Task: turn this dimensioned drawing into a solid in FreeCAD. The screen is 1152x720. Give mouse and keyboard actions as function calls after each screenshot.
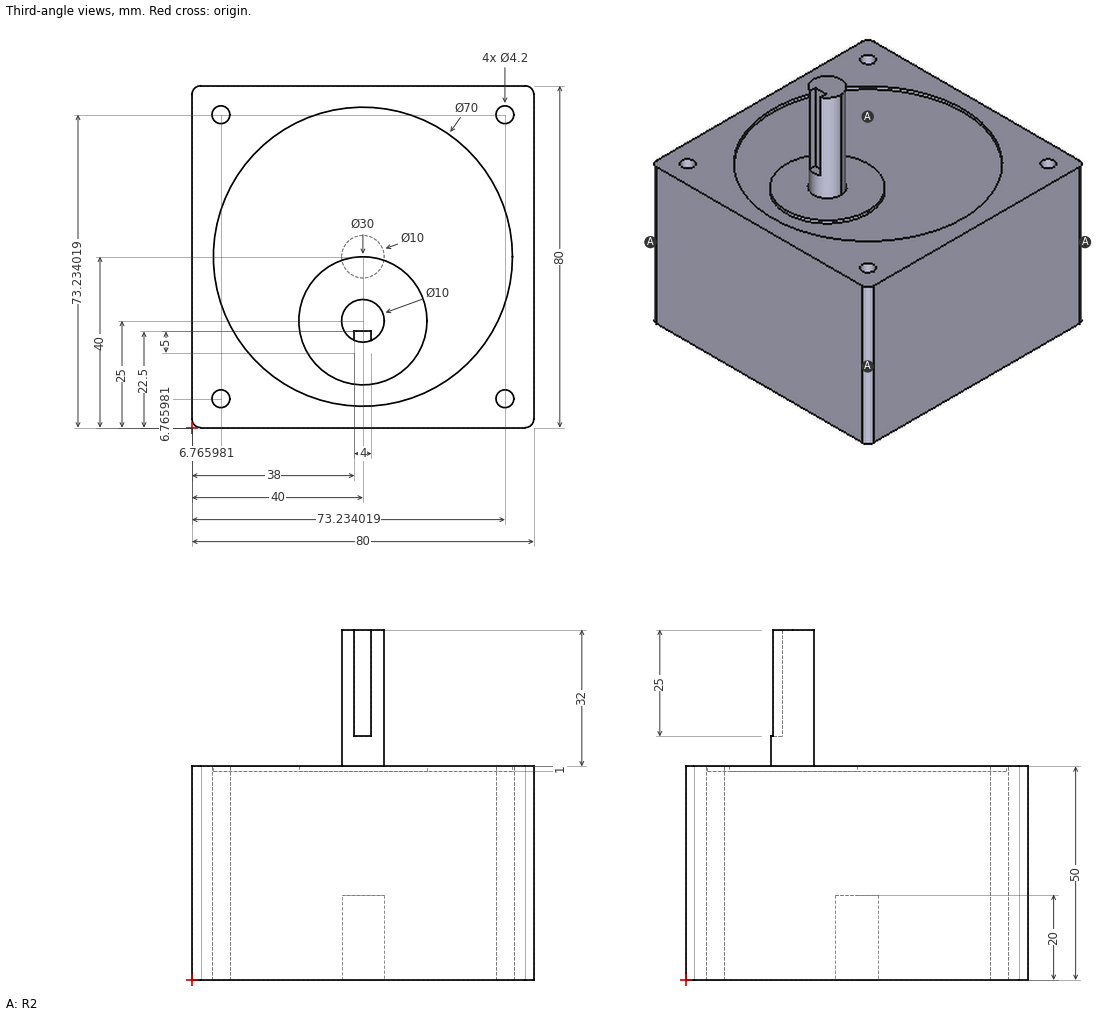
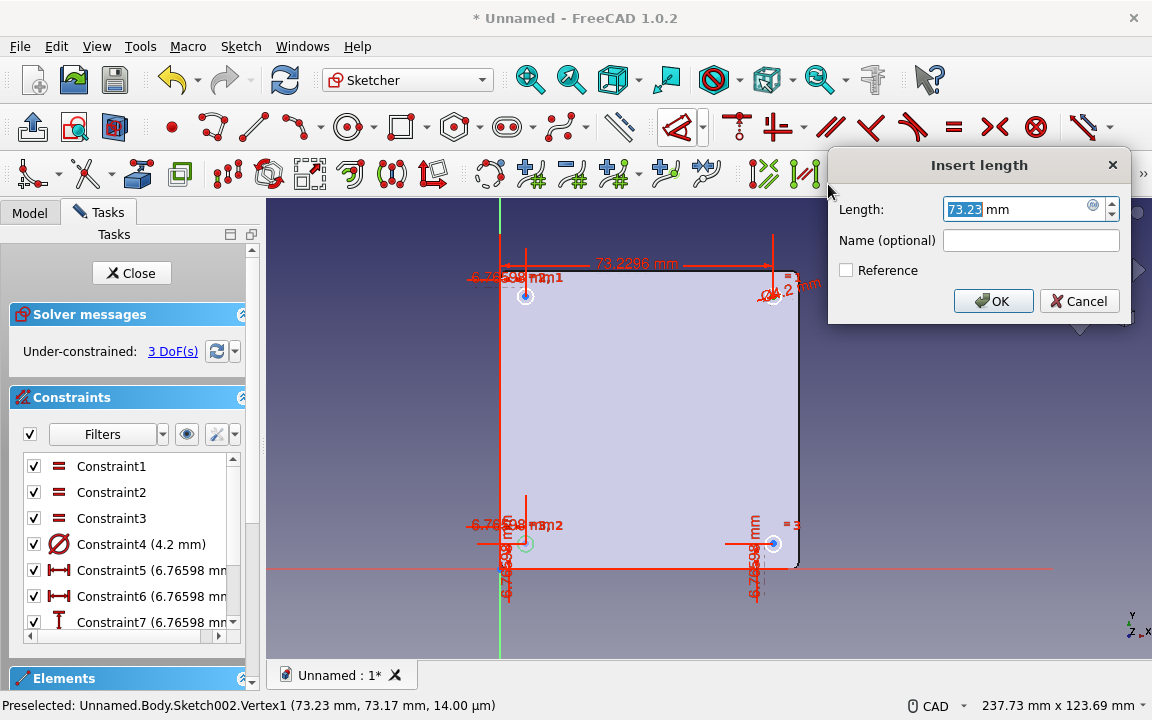
text(73.234019)
key(Return)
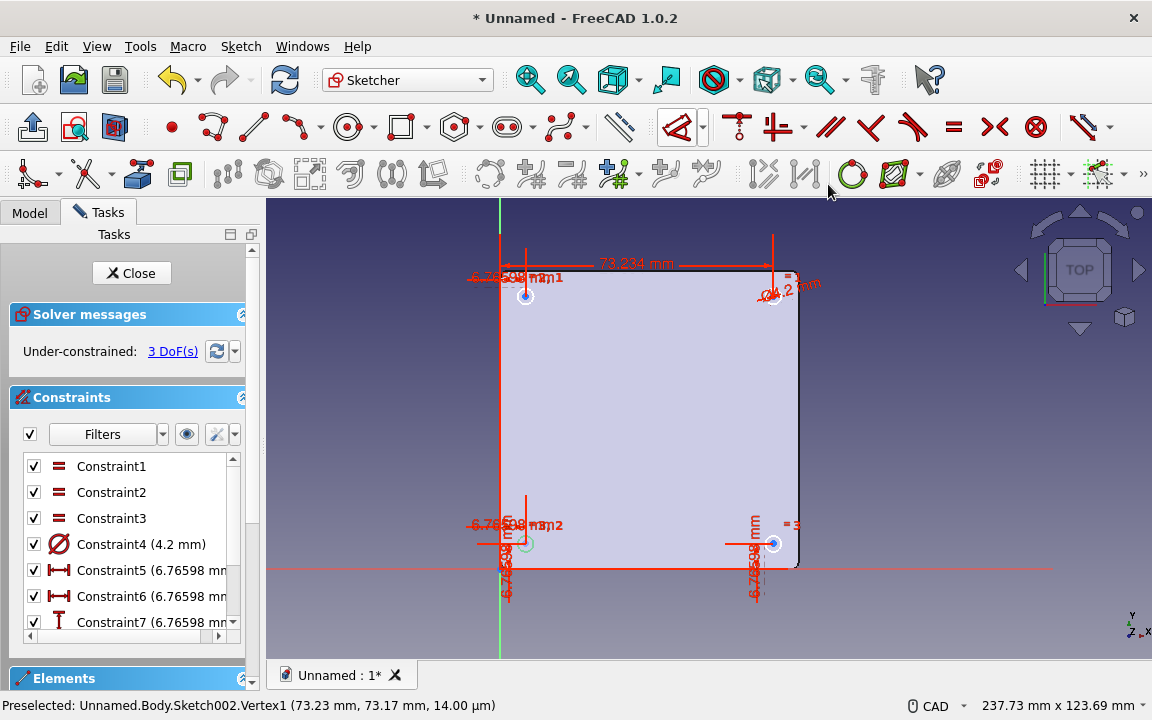
click(773, 296)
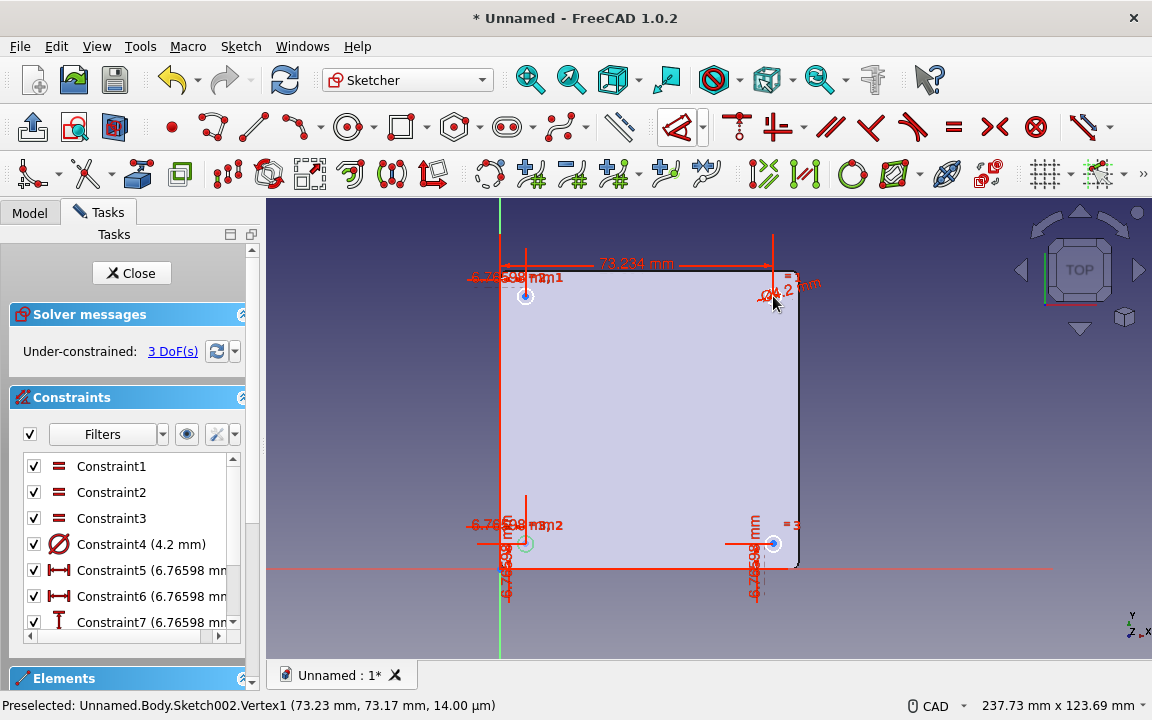
click(702, 128)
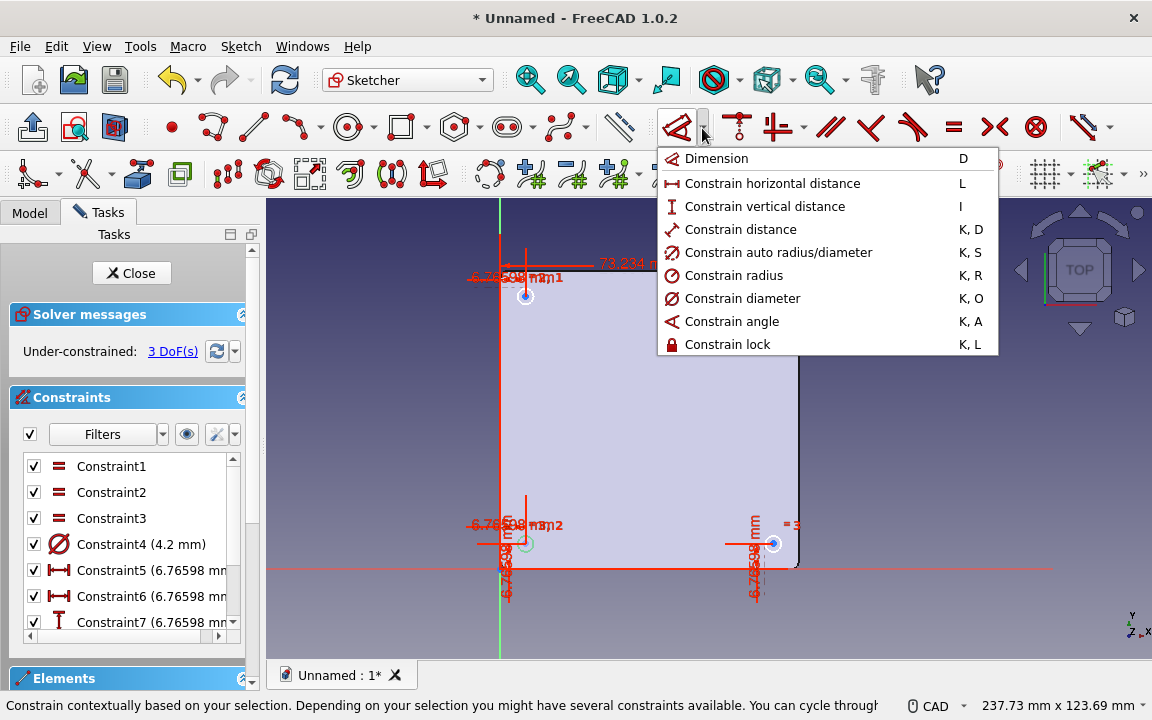
click(828, 206)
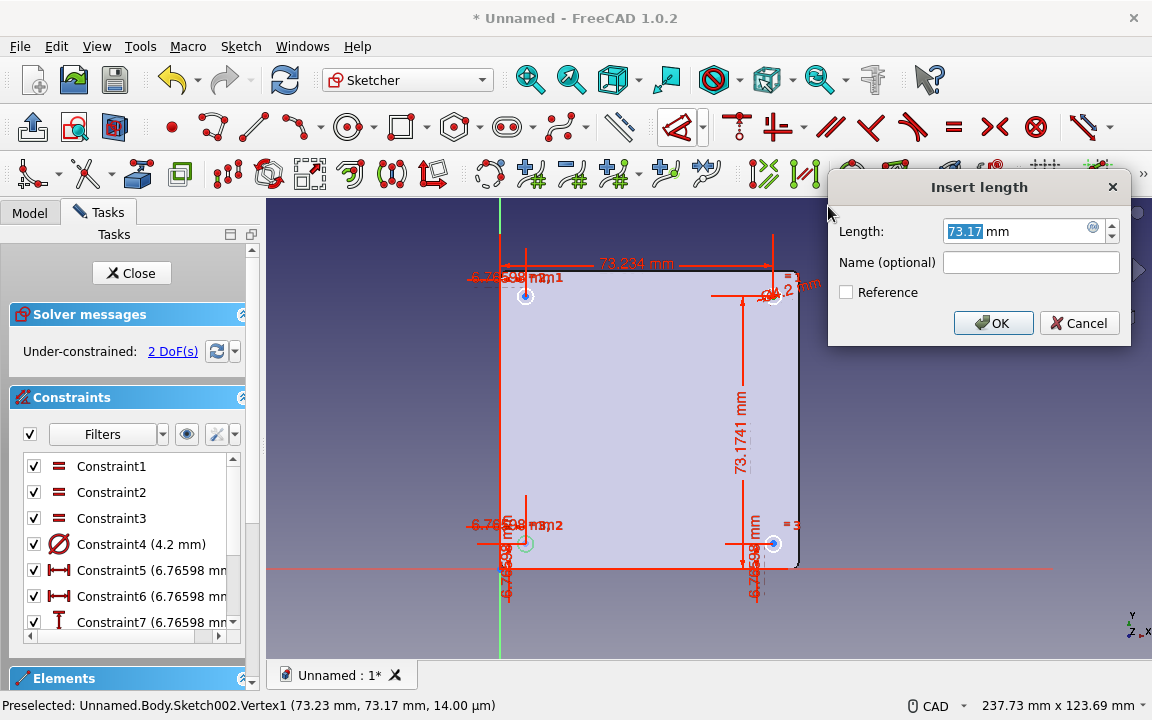
text(73.234019)
key(Return)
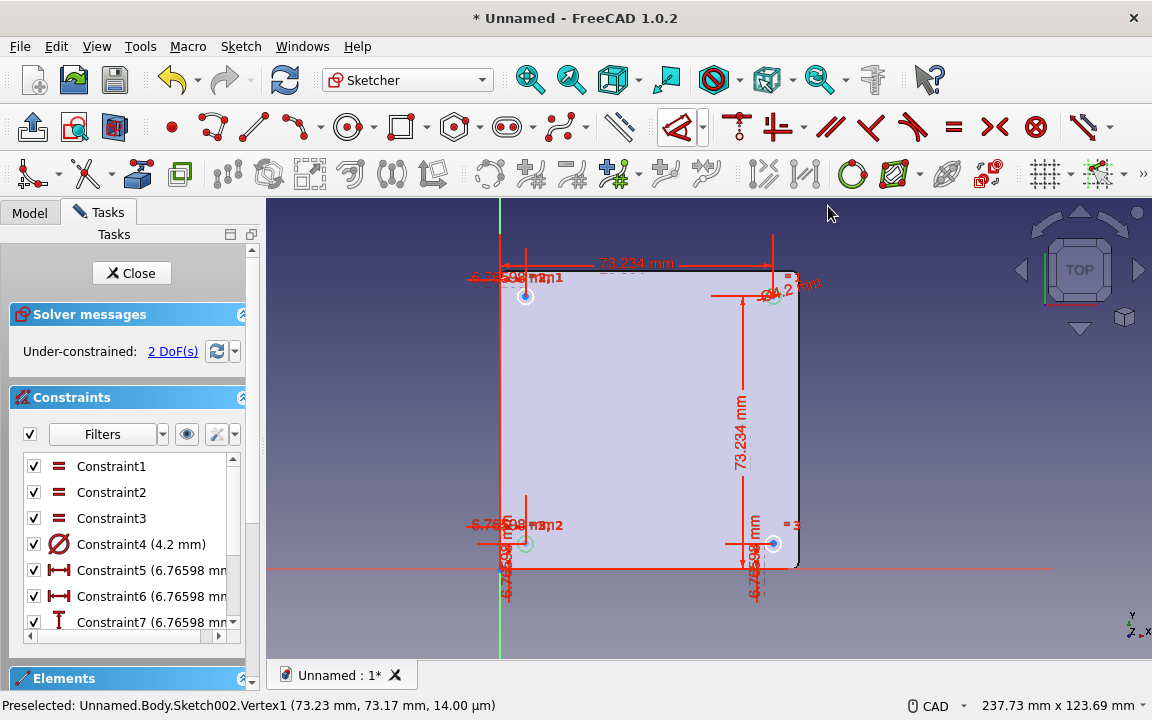
click(526, 296)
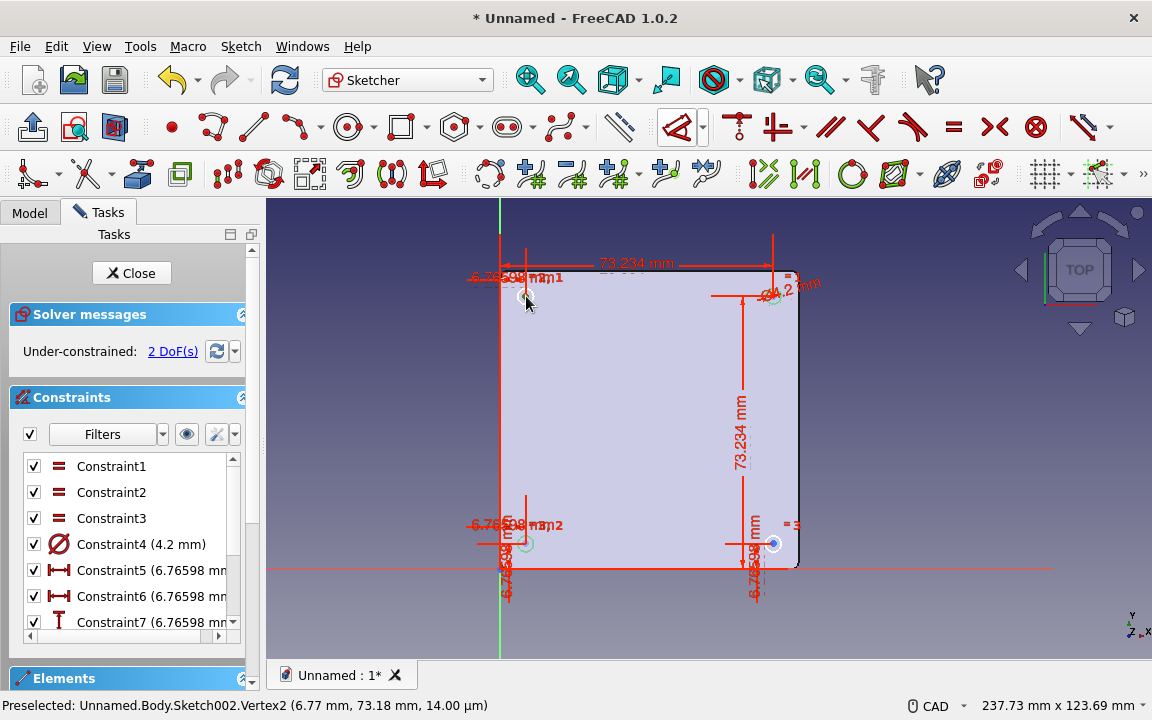
key(i)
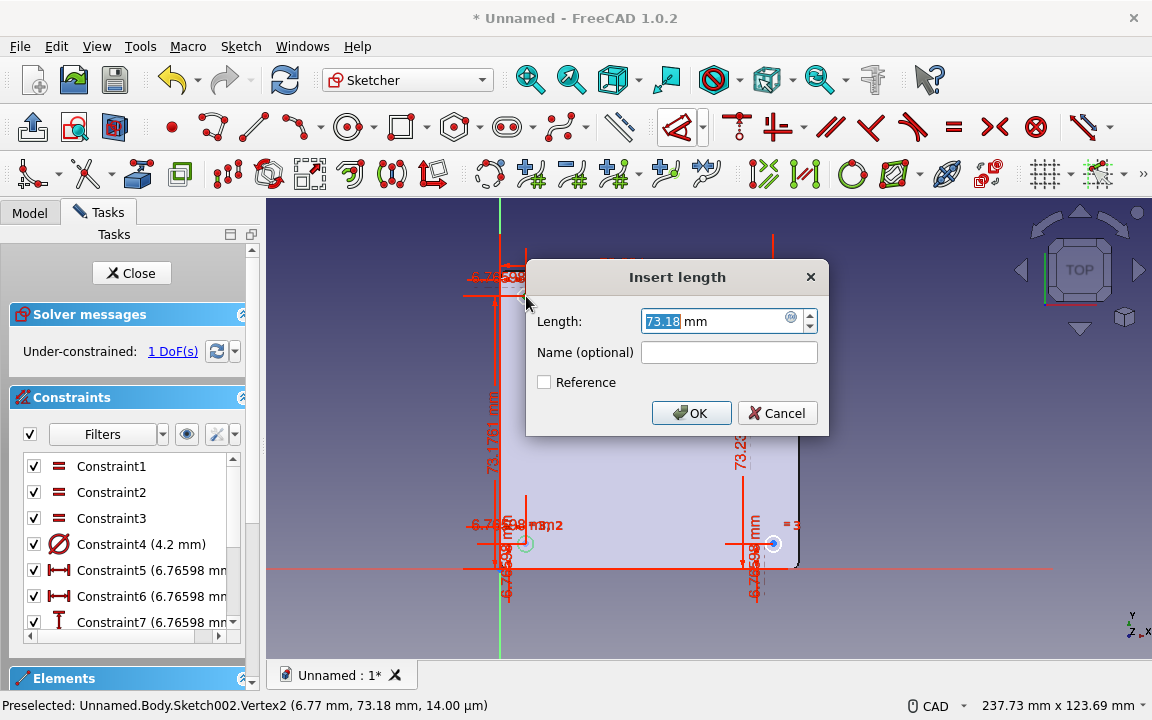
text(73.234019)
key(Return)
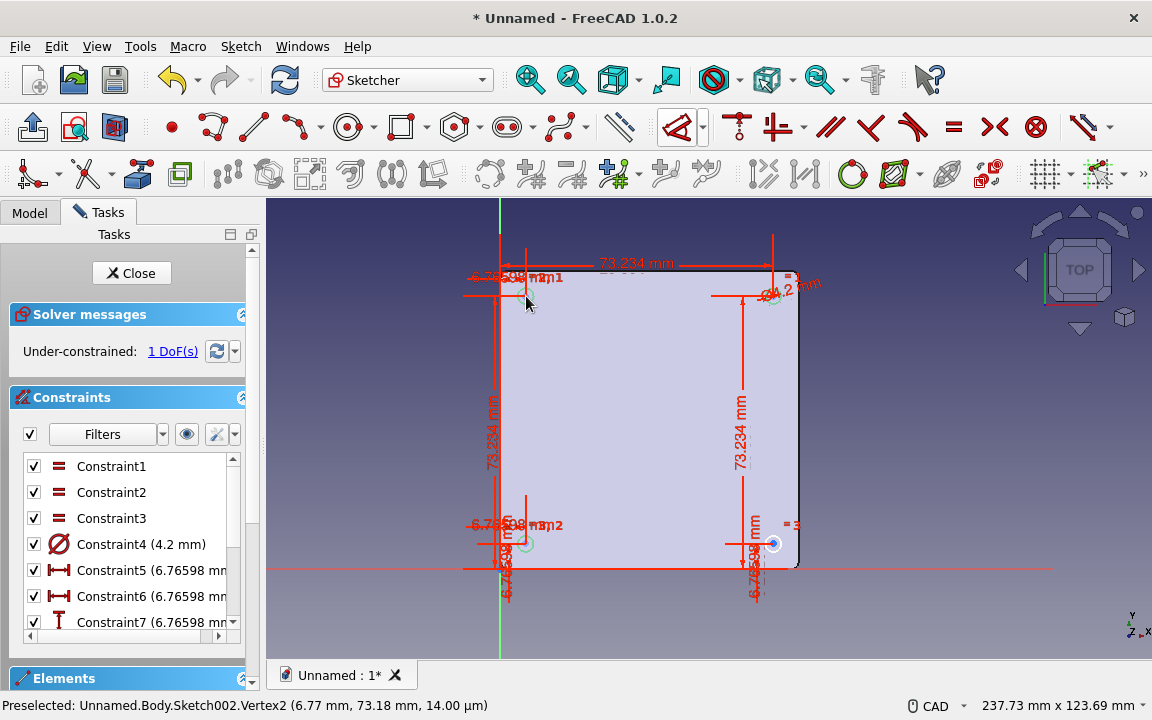
click(773, 544)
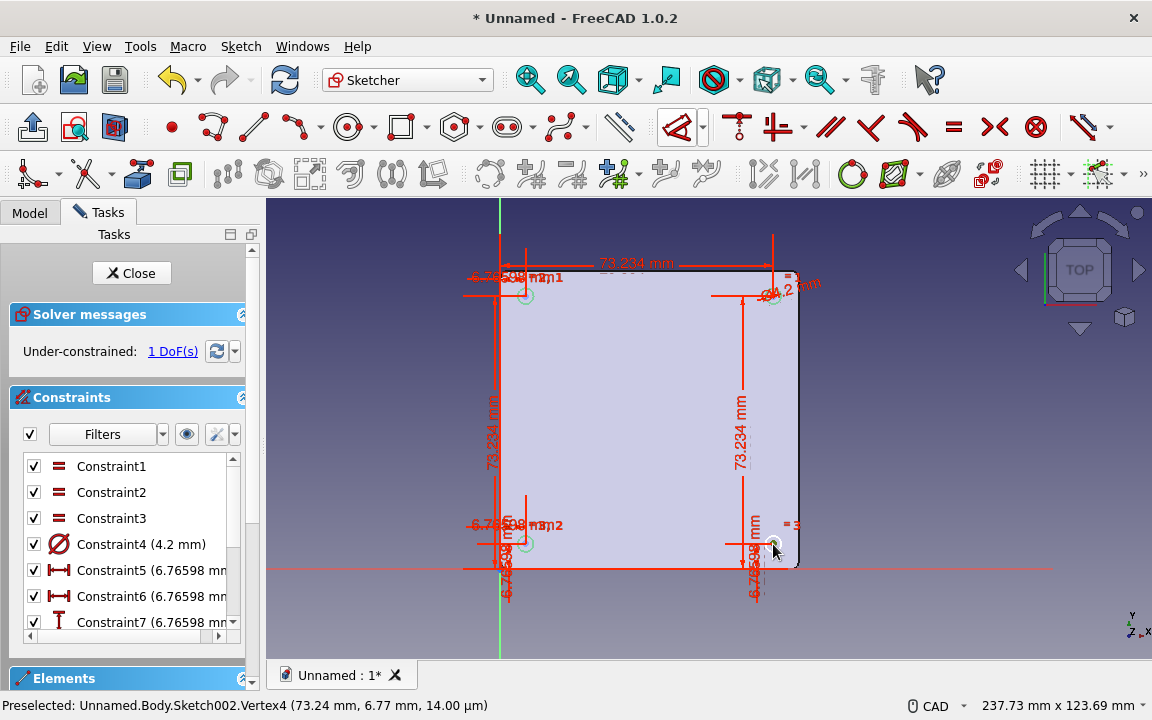
key(l)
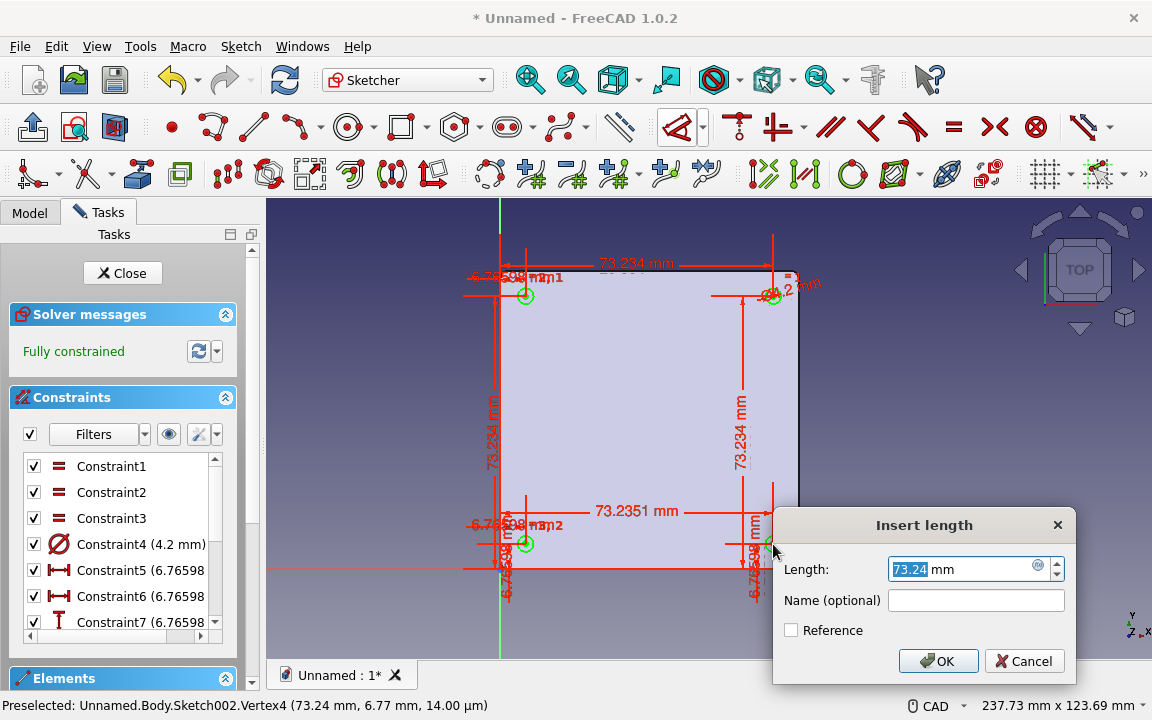
text(73.234019)
key(Return)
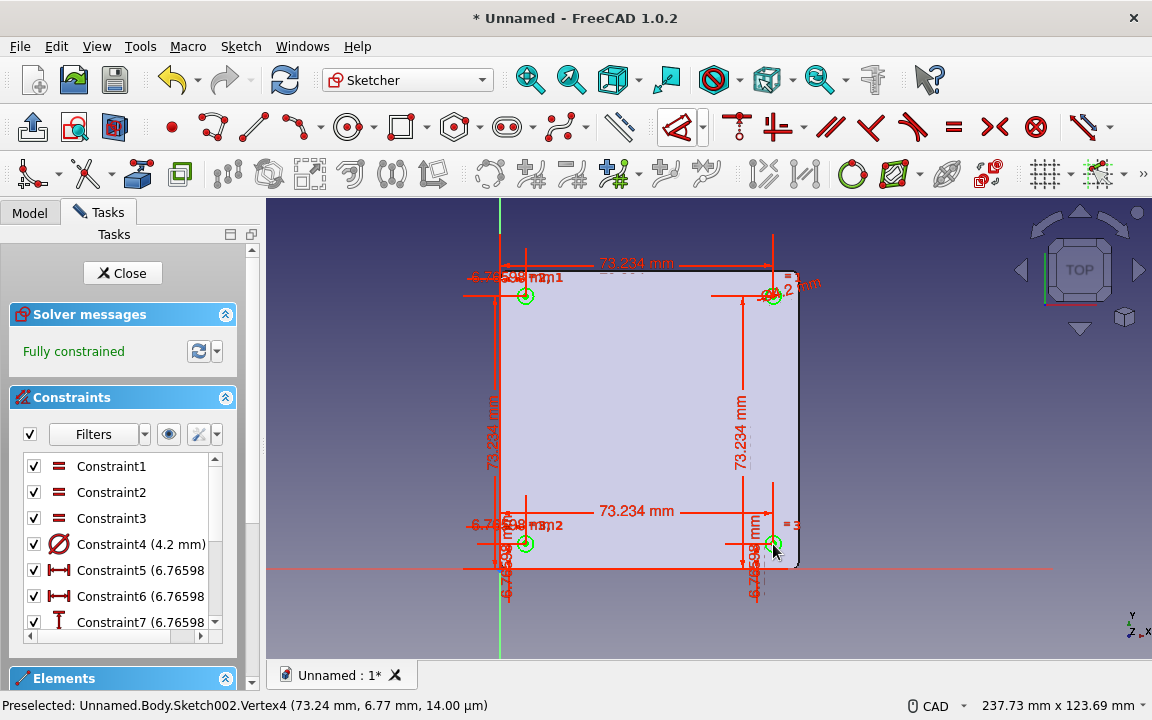
click(123, 273)